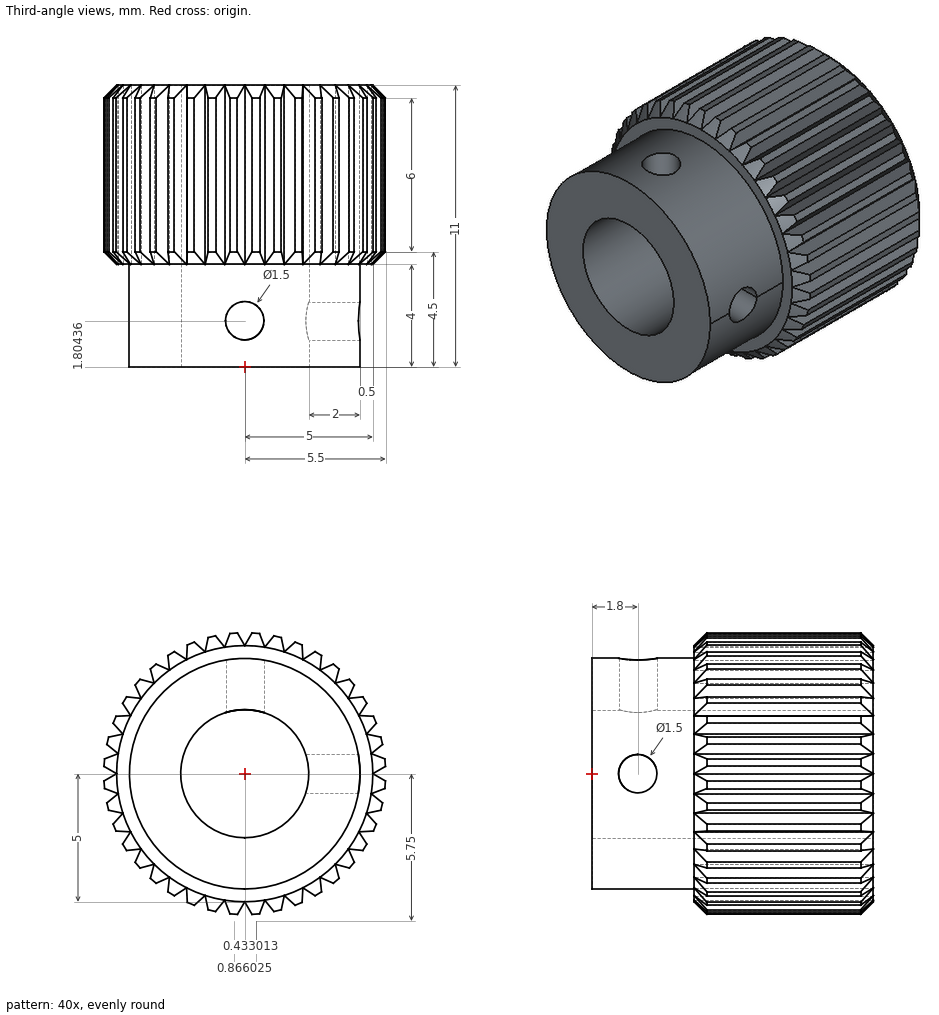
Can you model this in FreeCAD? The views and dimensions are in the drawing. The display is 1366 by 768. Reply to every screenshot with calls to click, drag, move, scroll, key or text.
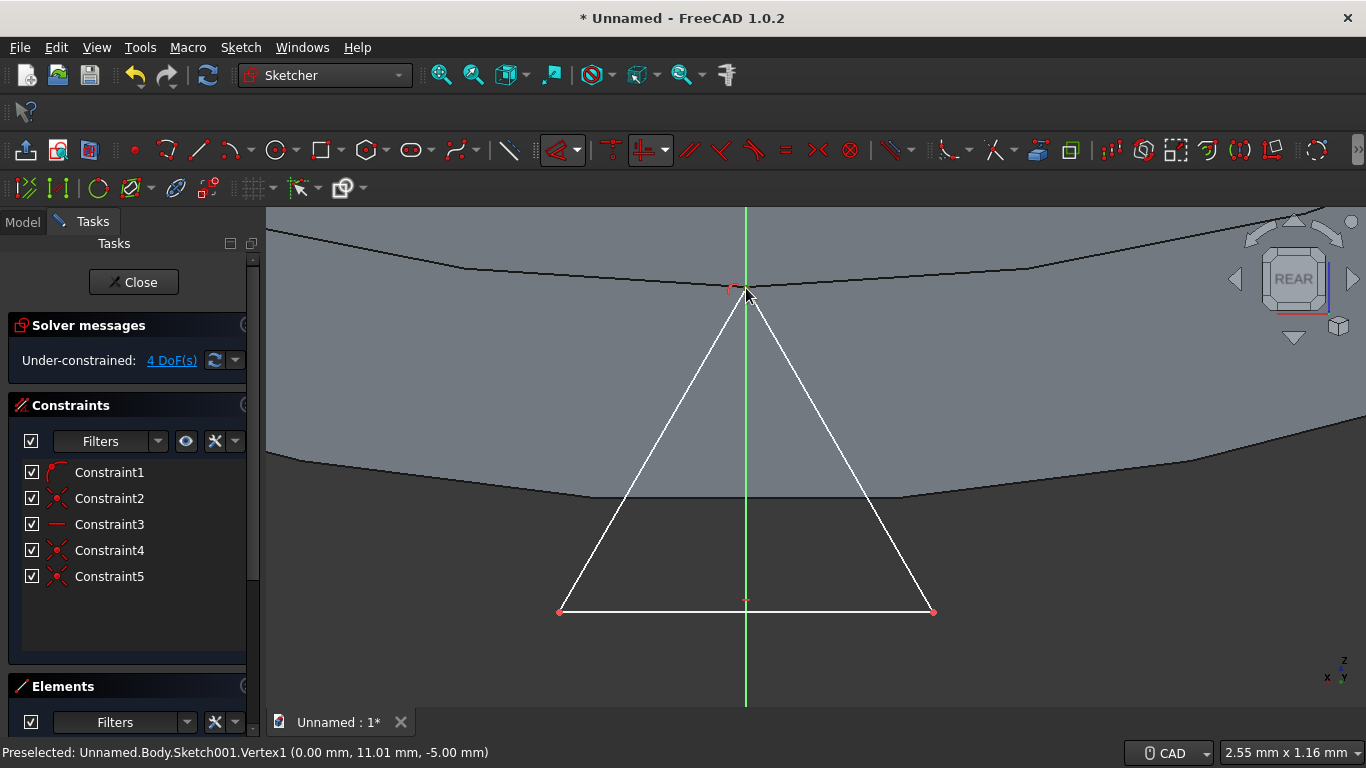
key(i)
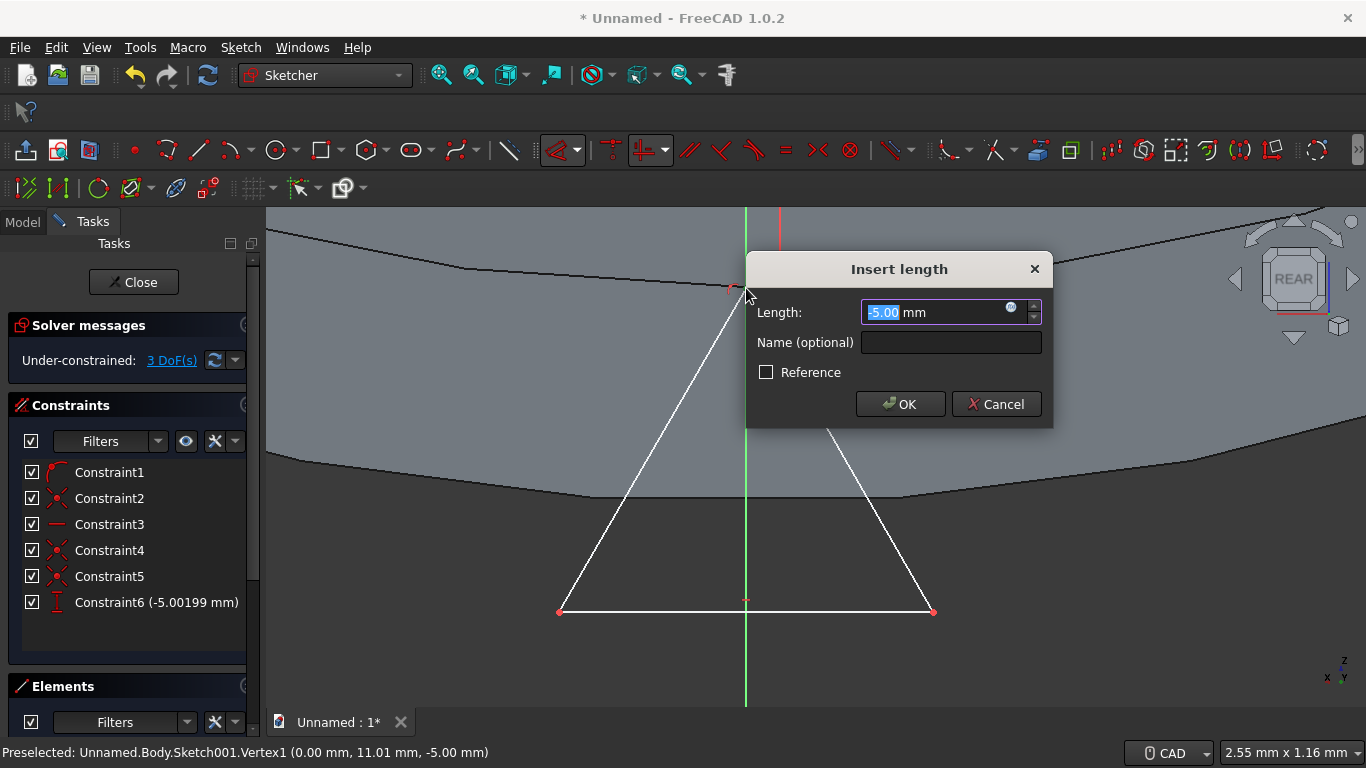
text(-5)
key(Return)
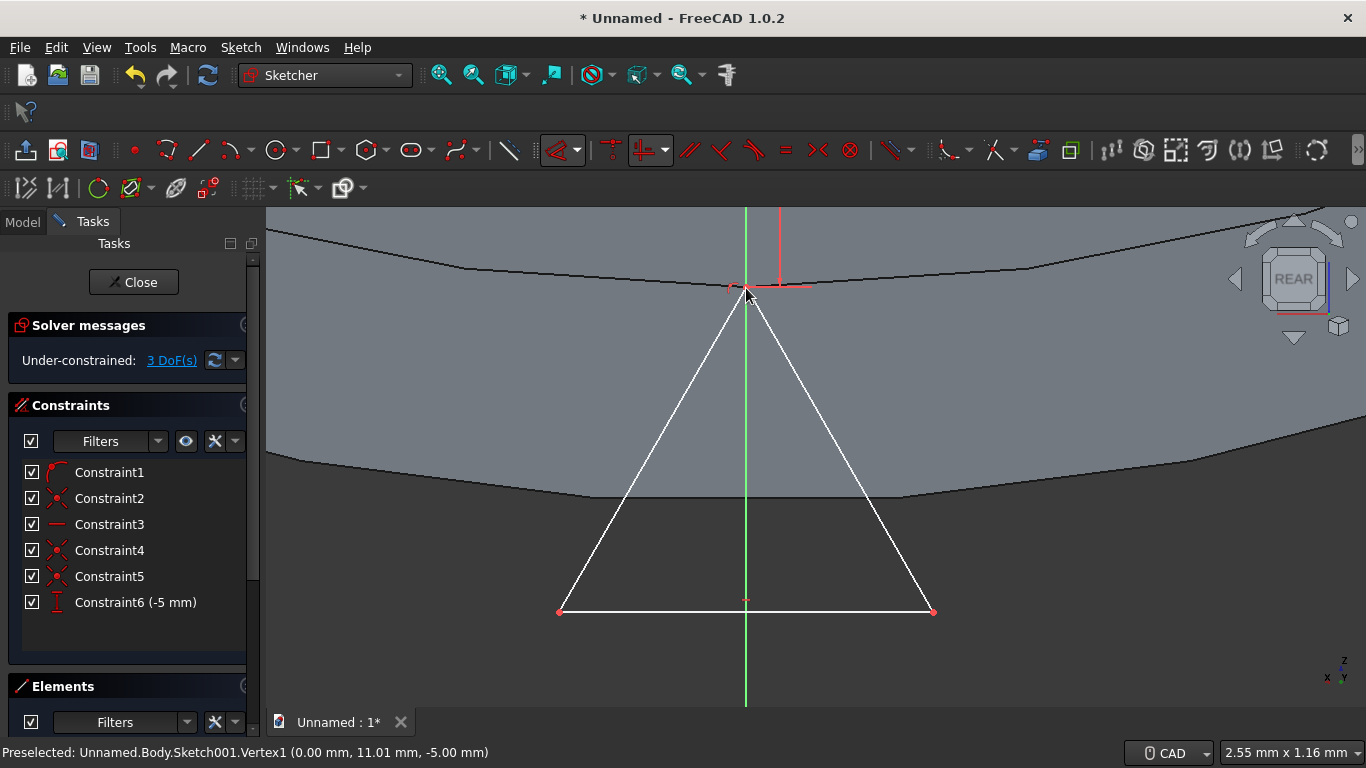
click(559, 612)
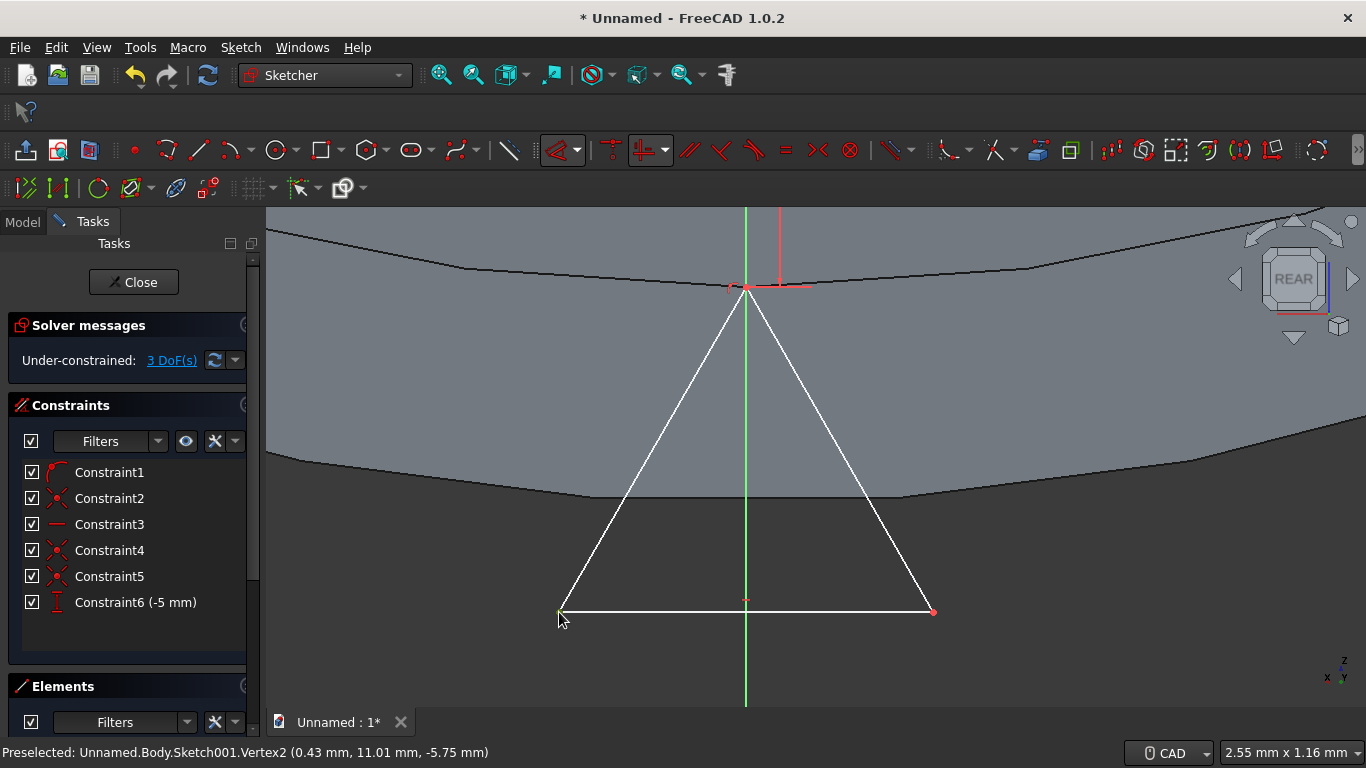
key(i)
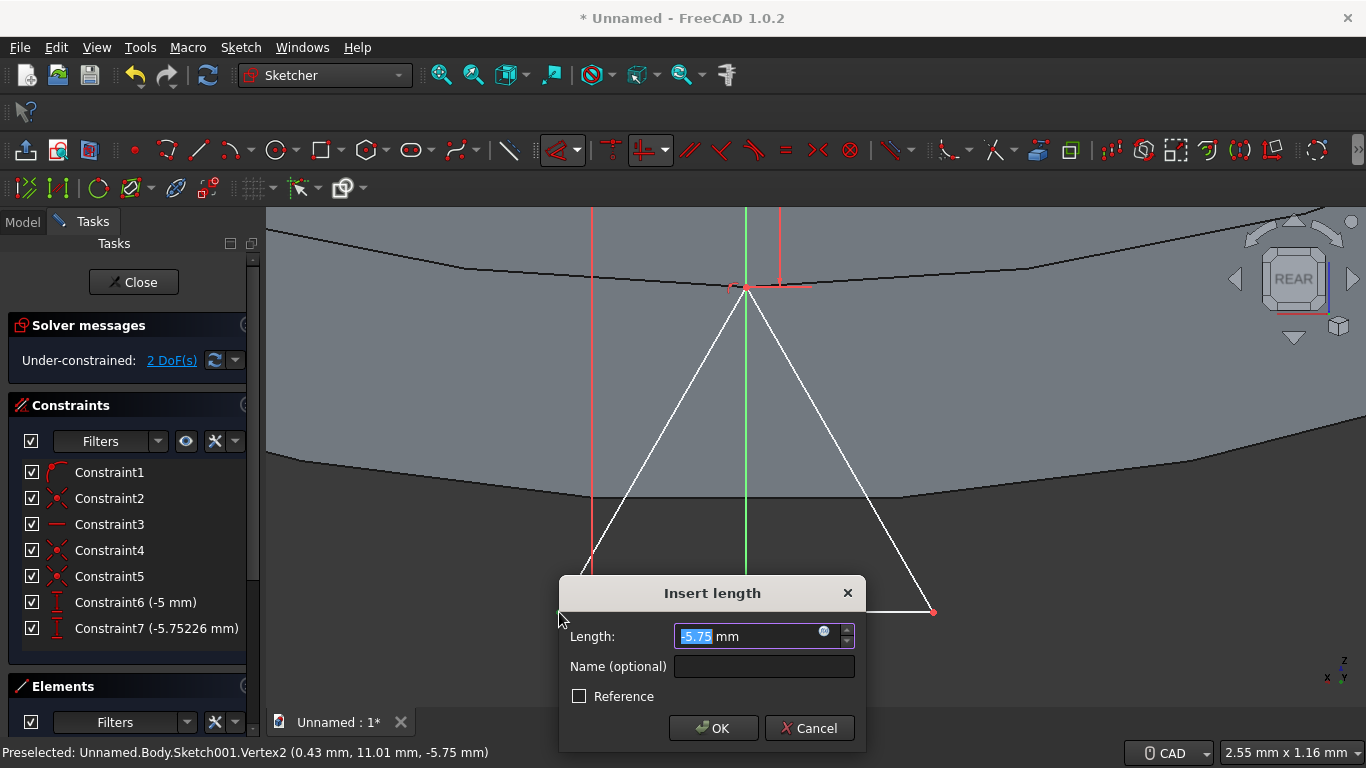
text(-5.75)
key(Return)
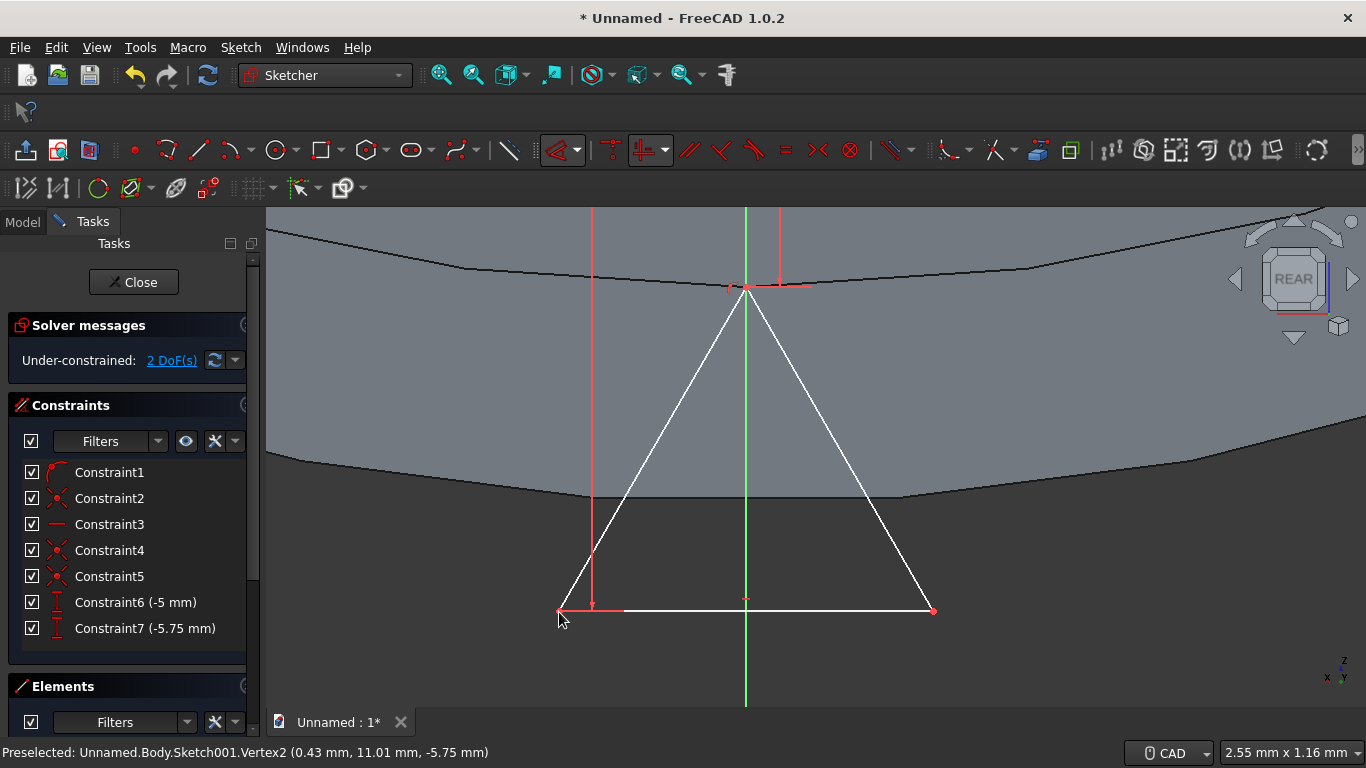
click(671, 611)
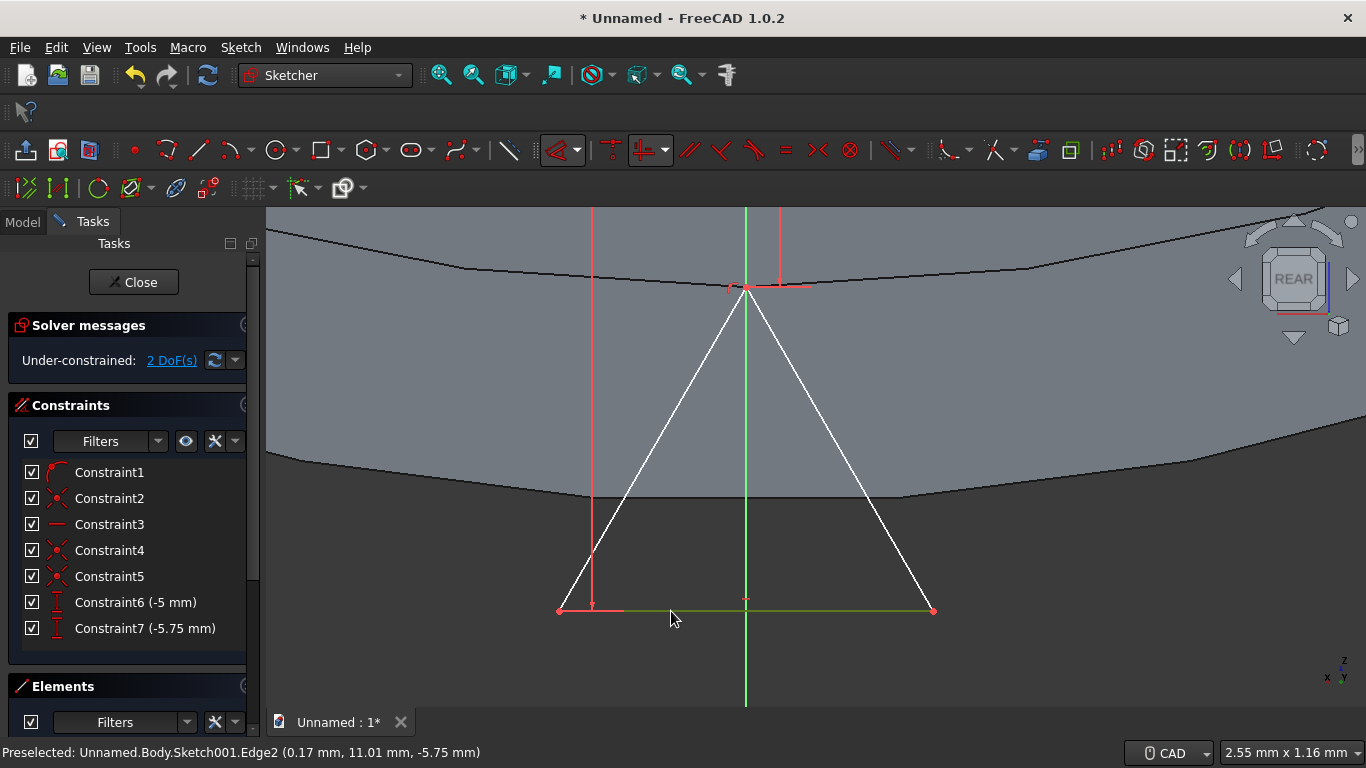
key(l)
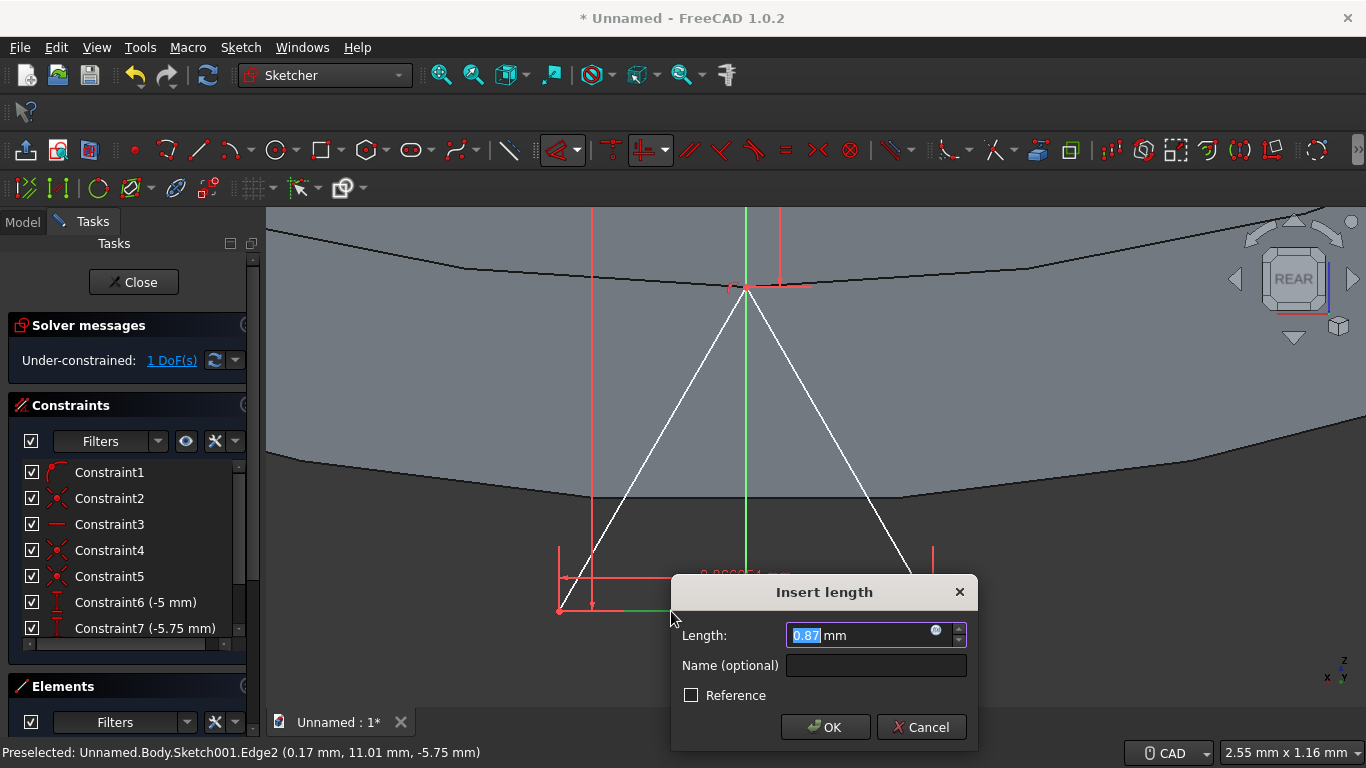
text(0.866025)
key(Return)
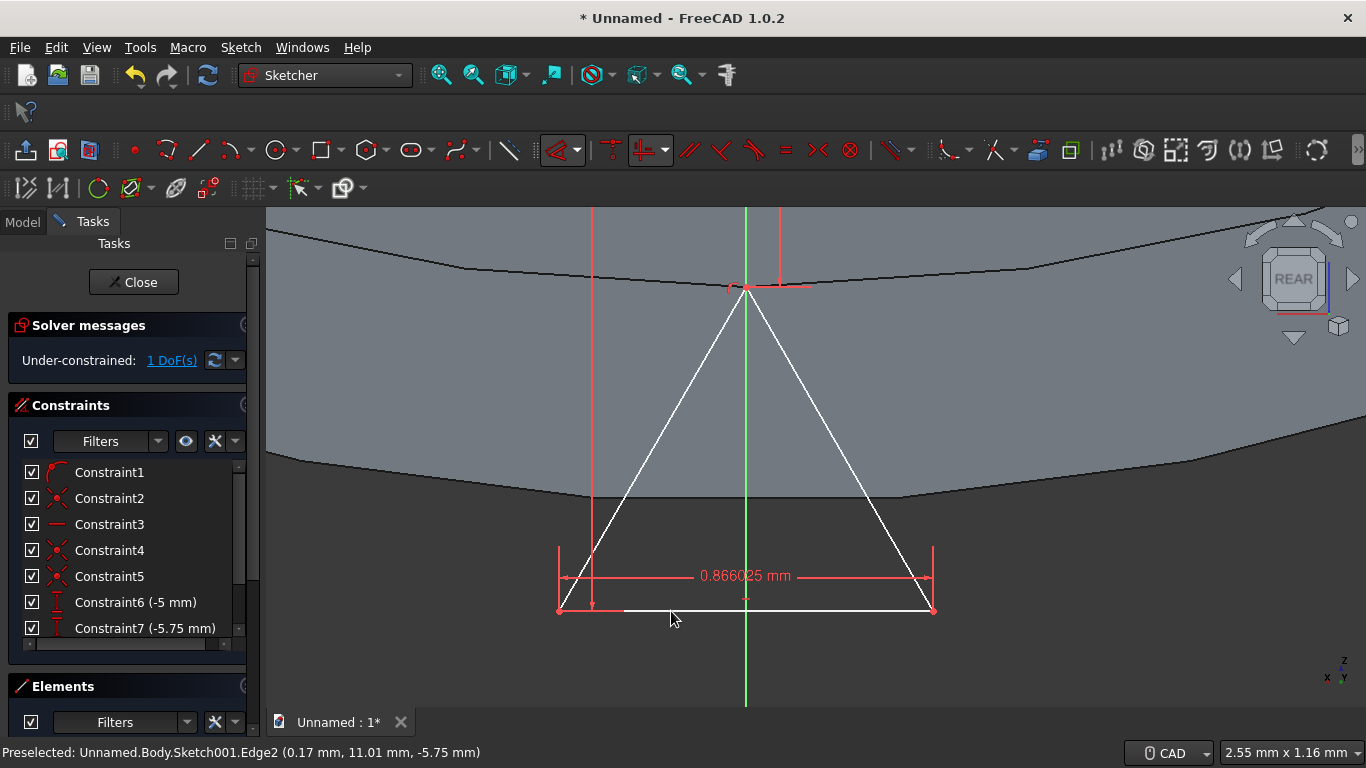
click(559, 611)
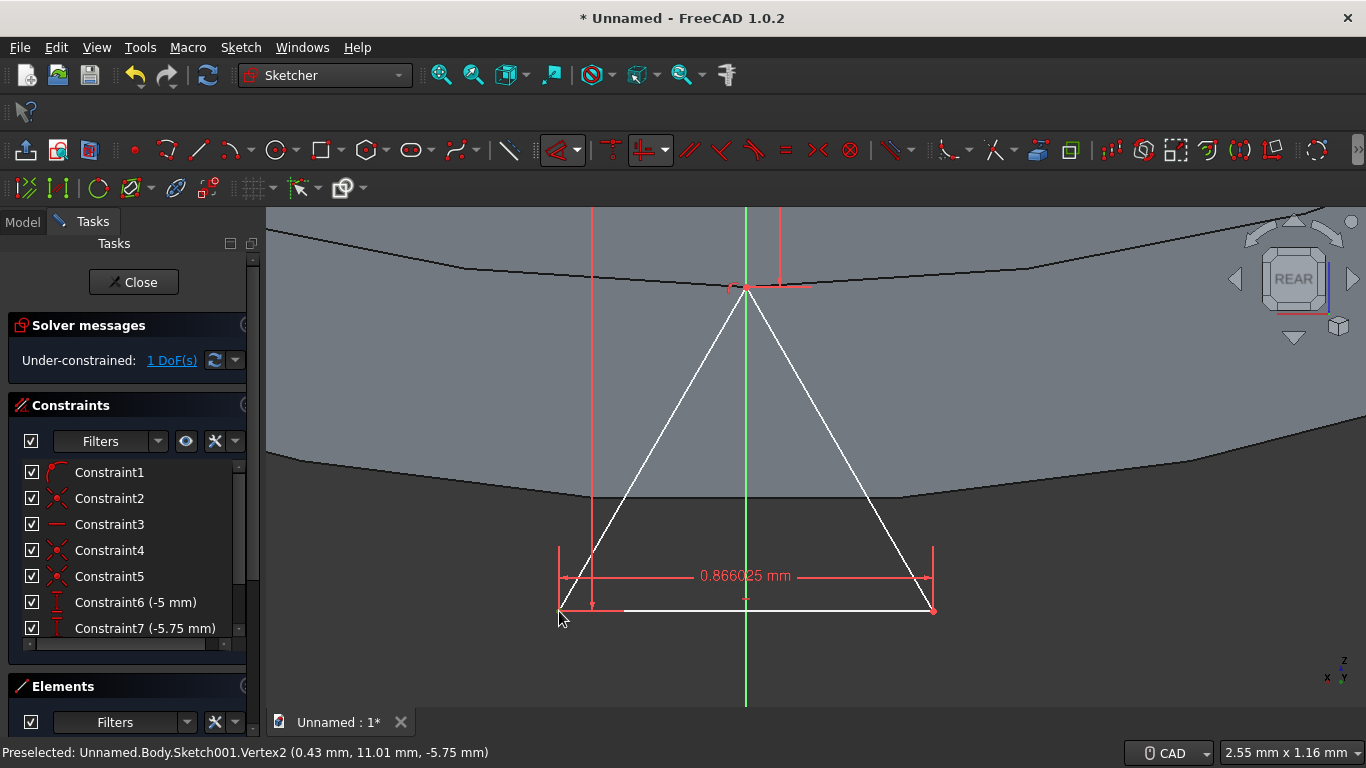
key(l)